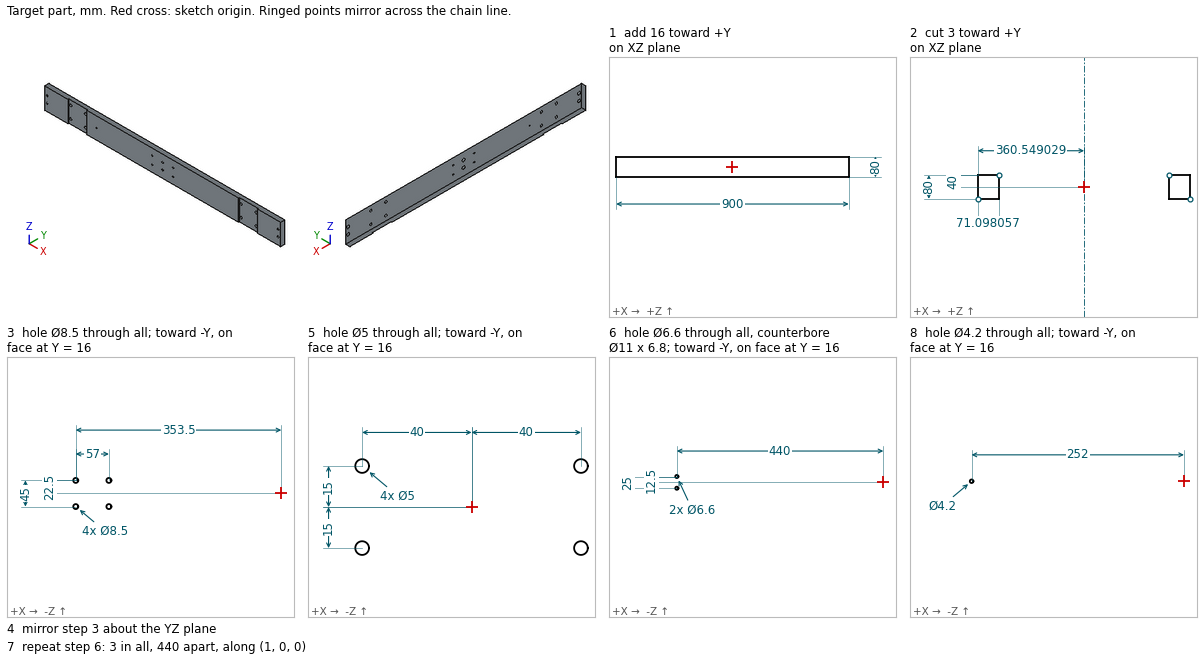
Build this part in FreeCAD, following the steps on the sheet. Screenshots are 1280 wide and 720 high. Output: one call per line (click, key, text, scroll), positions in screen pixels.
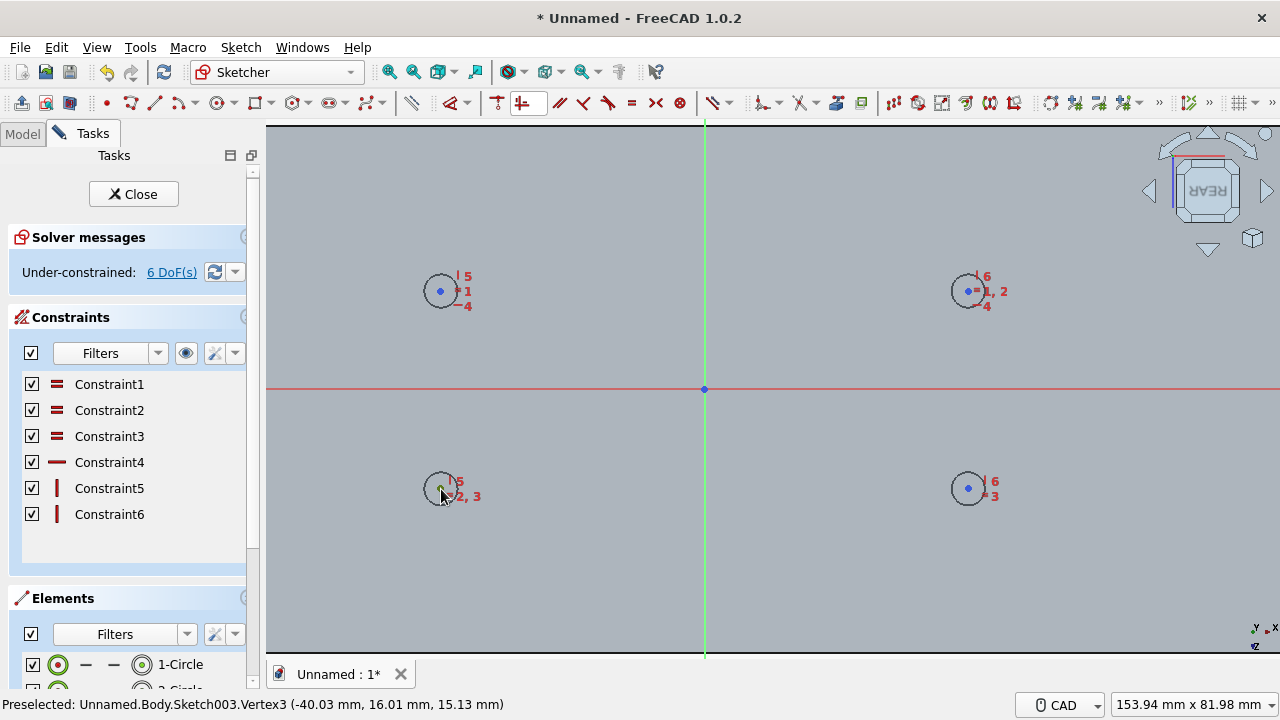
click(968, 489)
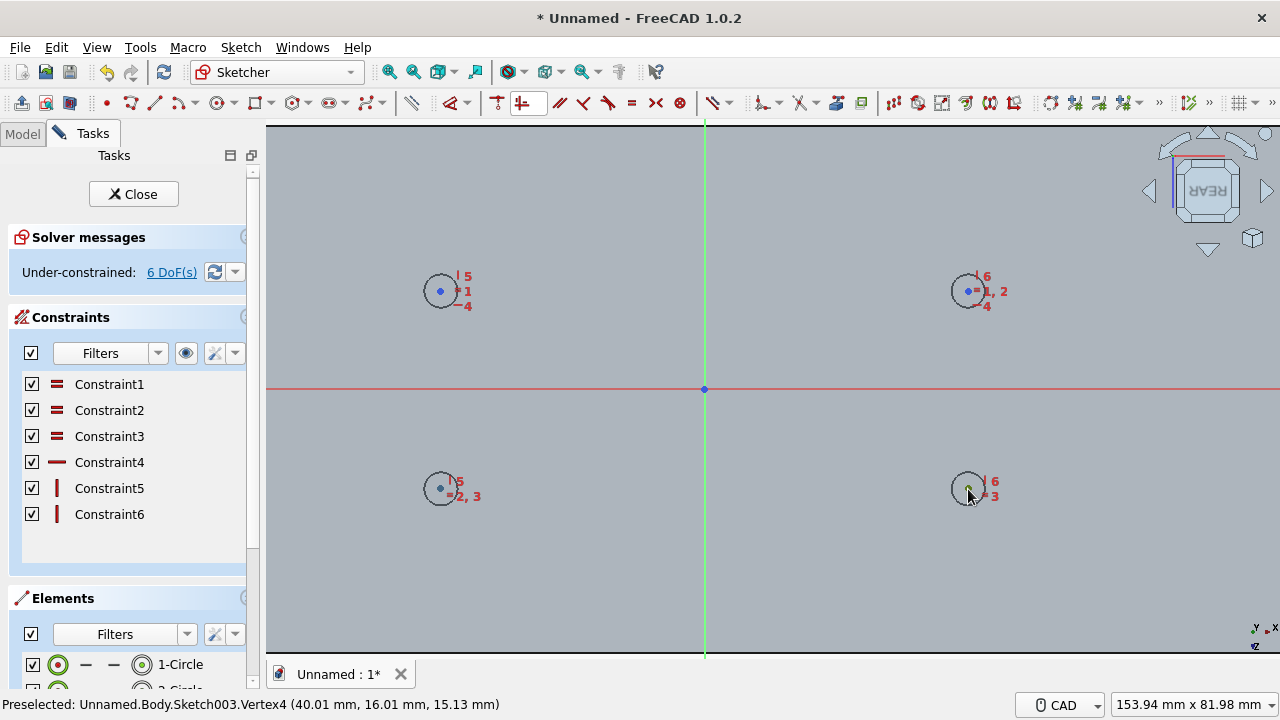
key(h)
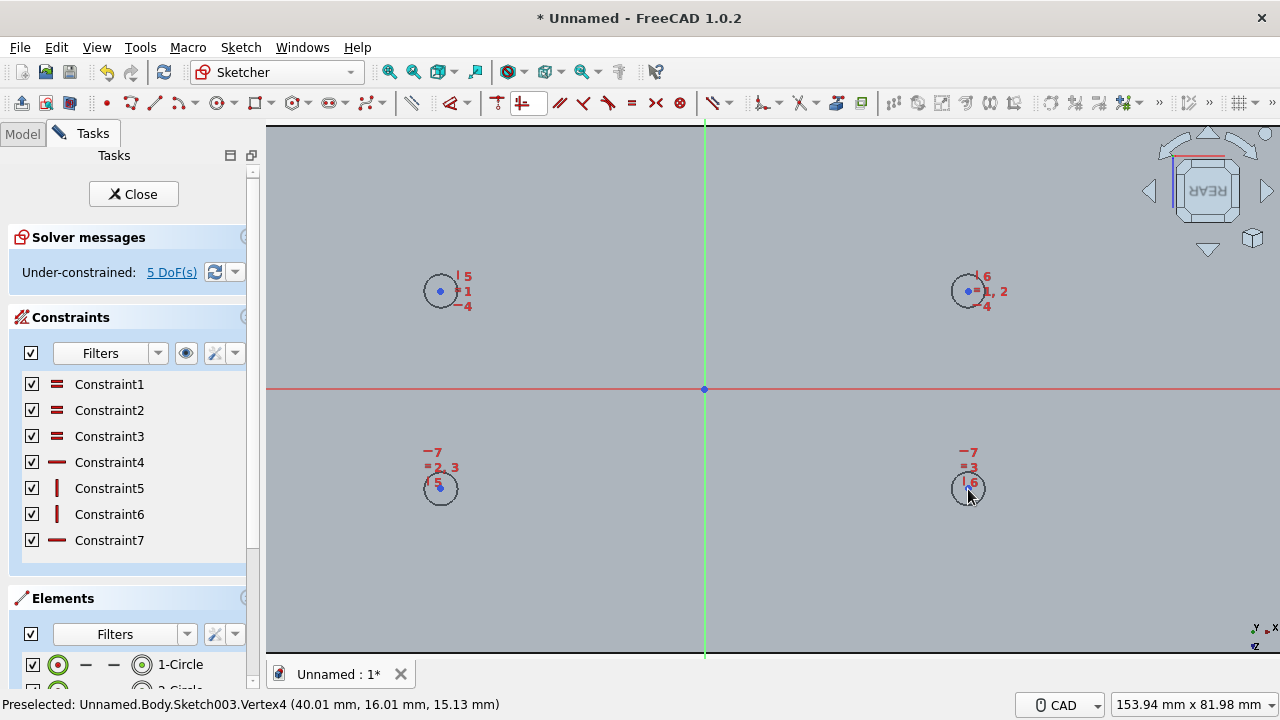
click(450, 104)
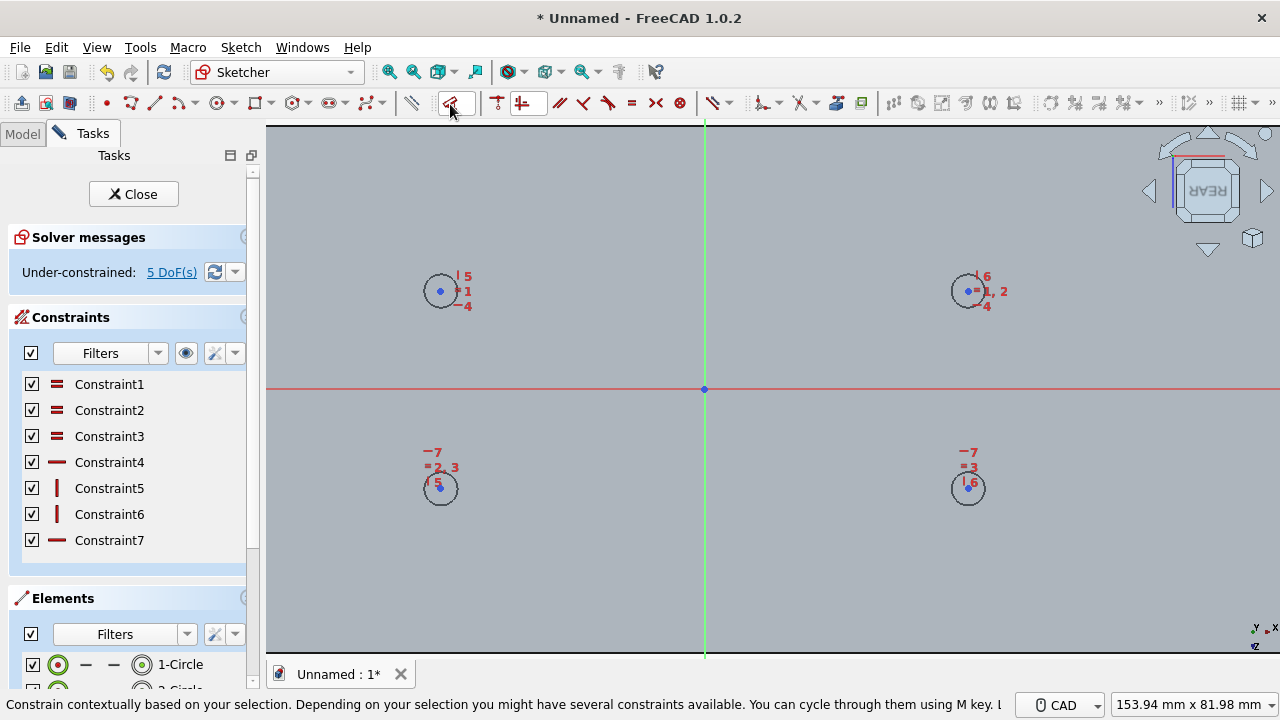
click(453, 279)
click(476, 256)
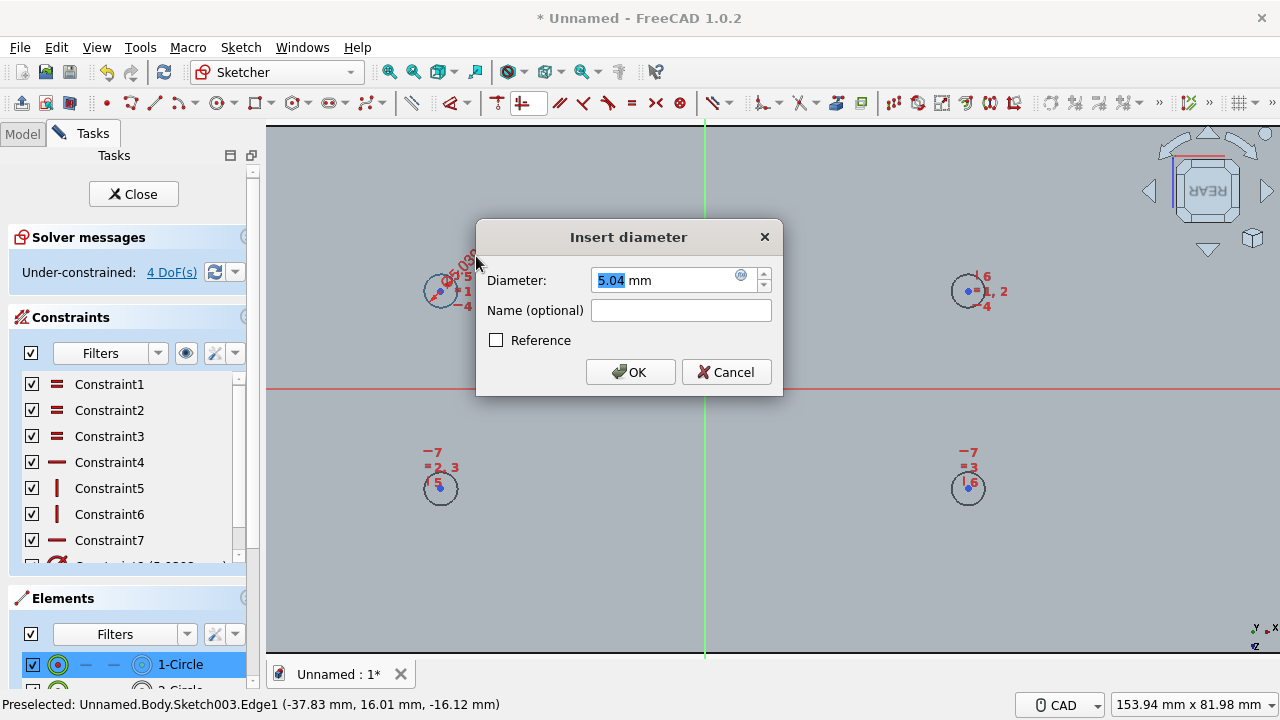
text(5)
key(Return)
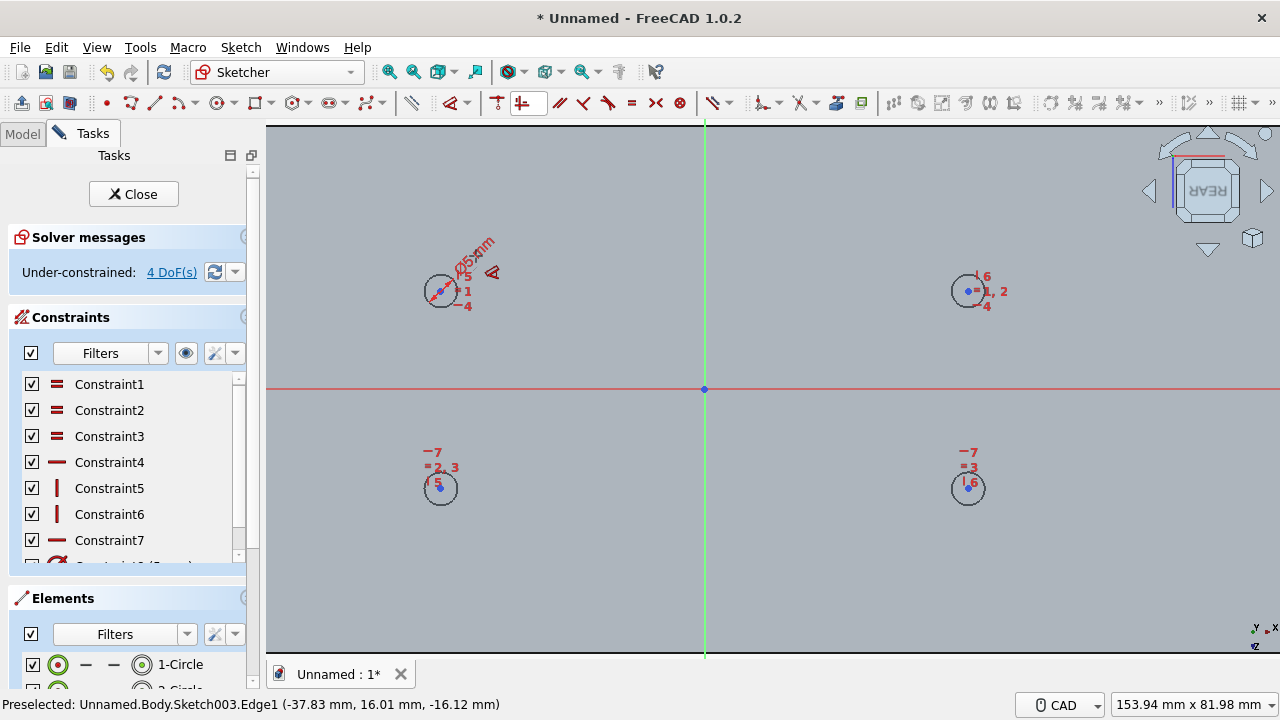
click(441, 291)
click(573, 257)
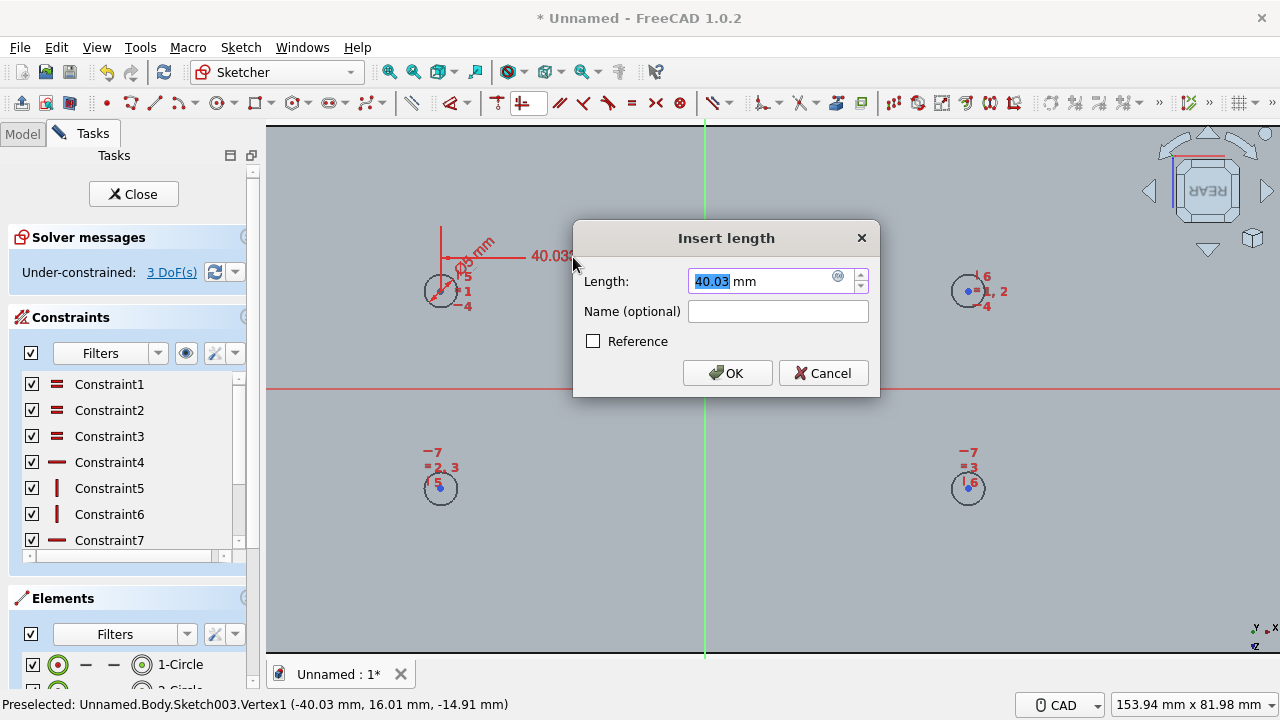
text(40)
key(Return)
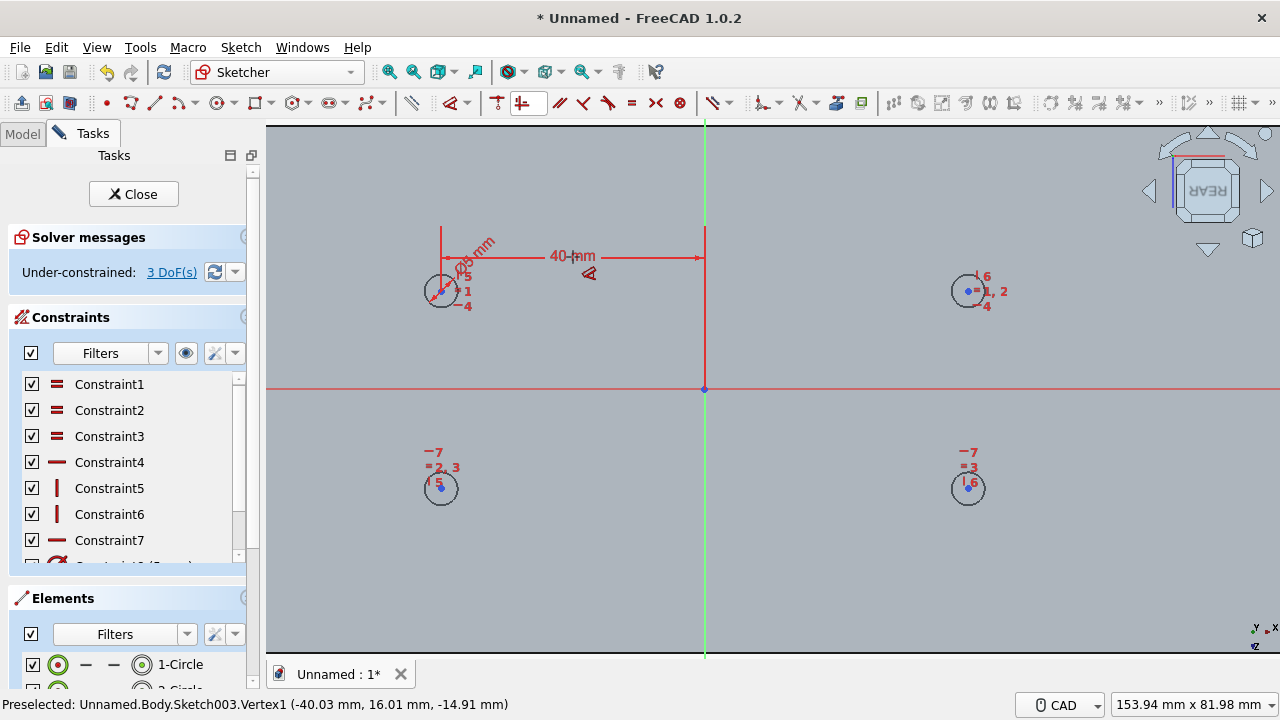
click(441, 291)
click(407, 340)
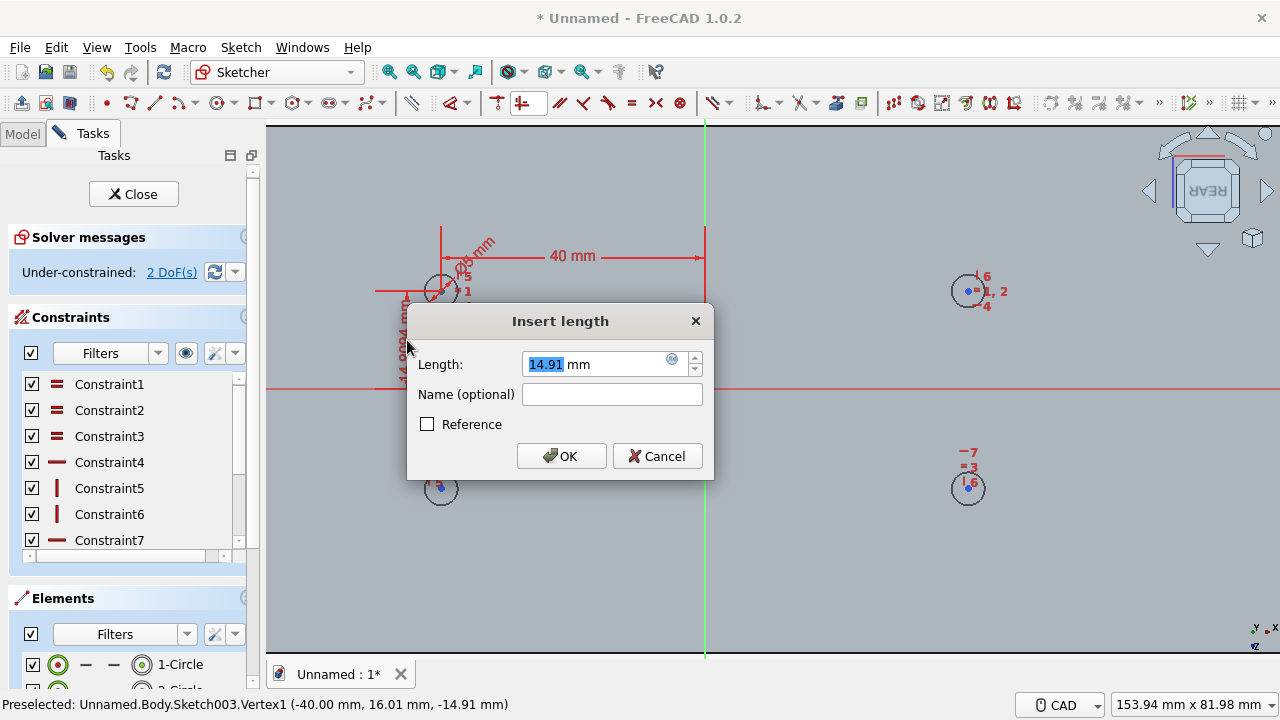
text(15)
key(Return)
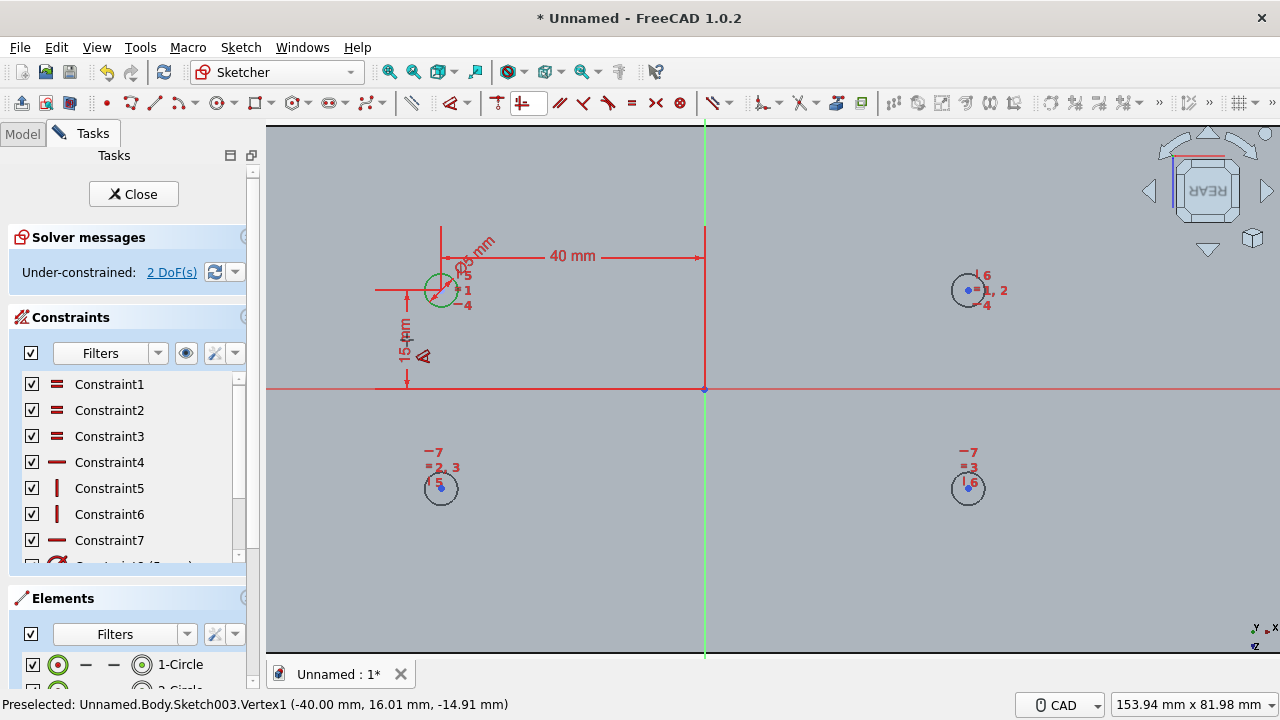
click(968, 290)
click(836, 256)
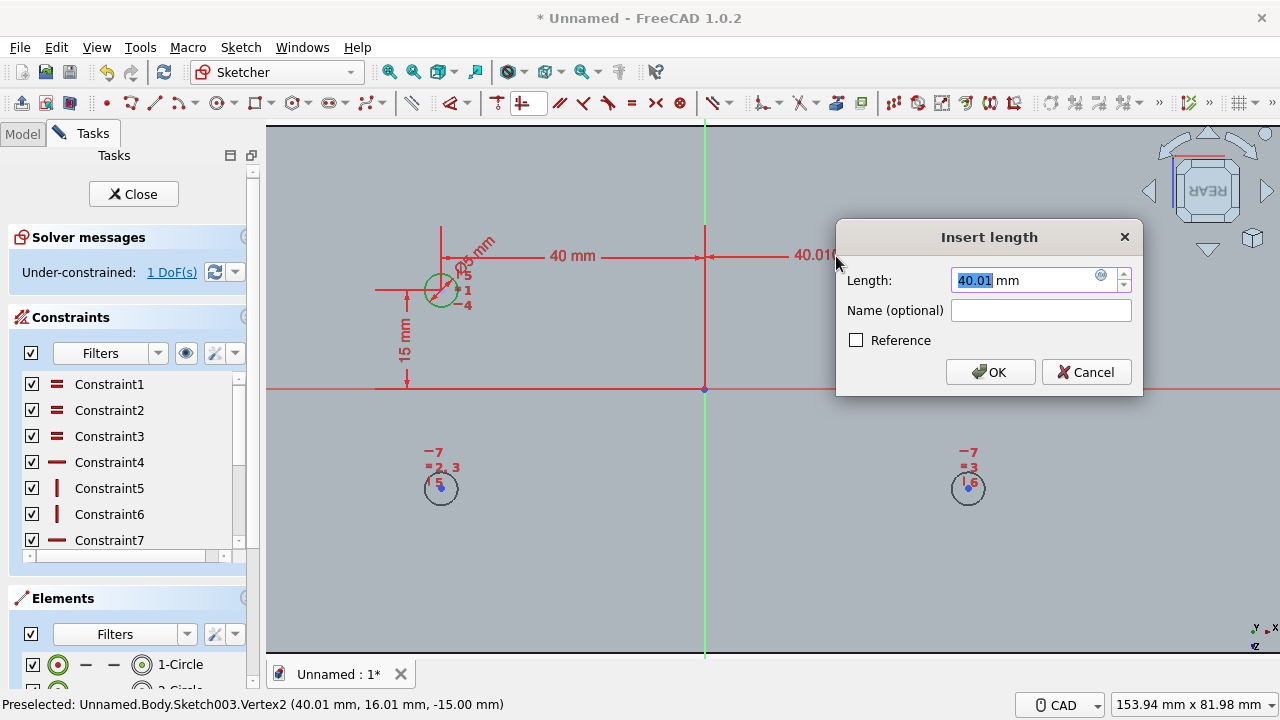
text(40)
key(Return)